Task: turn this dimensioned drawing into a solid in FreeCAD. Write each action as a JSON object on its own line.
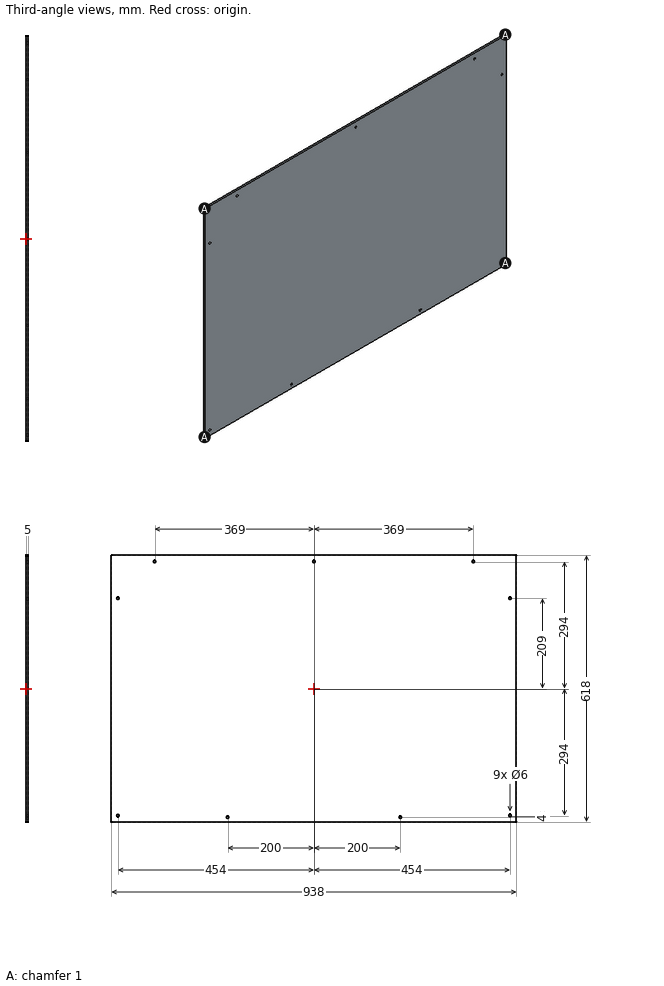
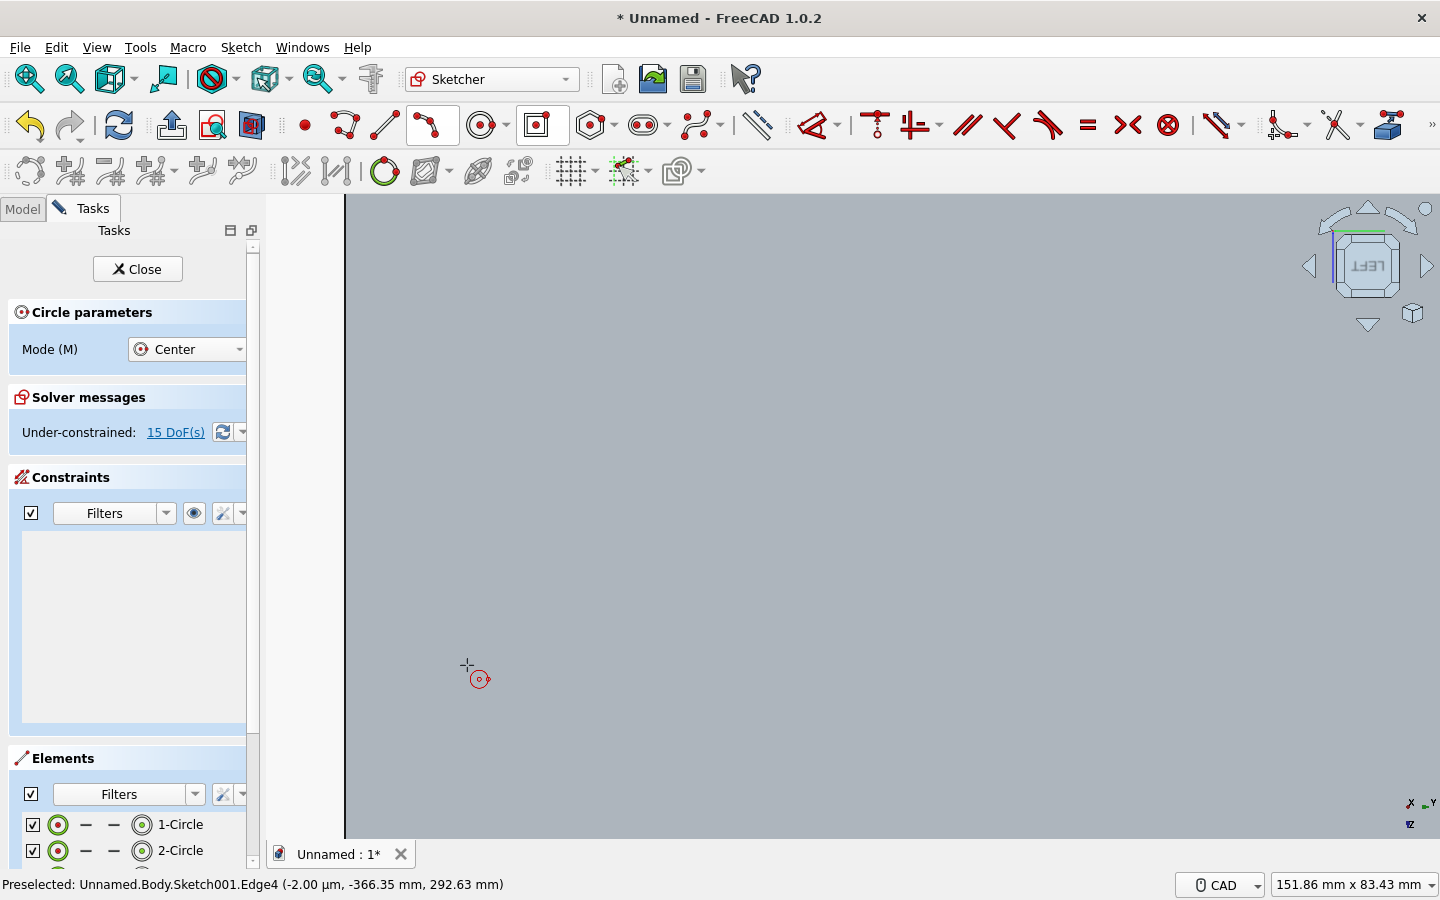
{"action": "scroll", "coordinate": [467, 665], "scroll_direction": "down", "scroll_amount": 12}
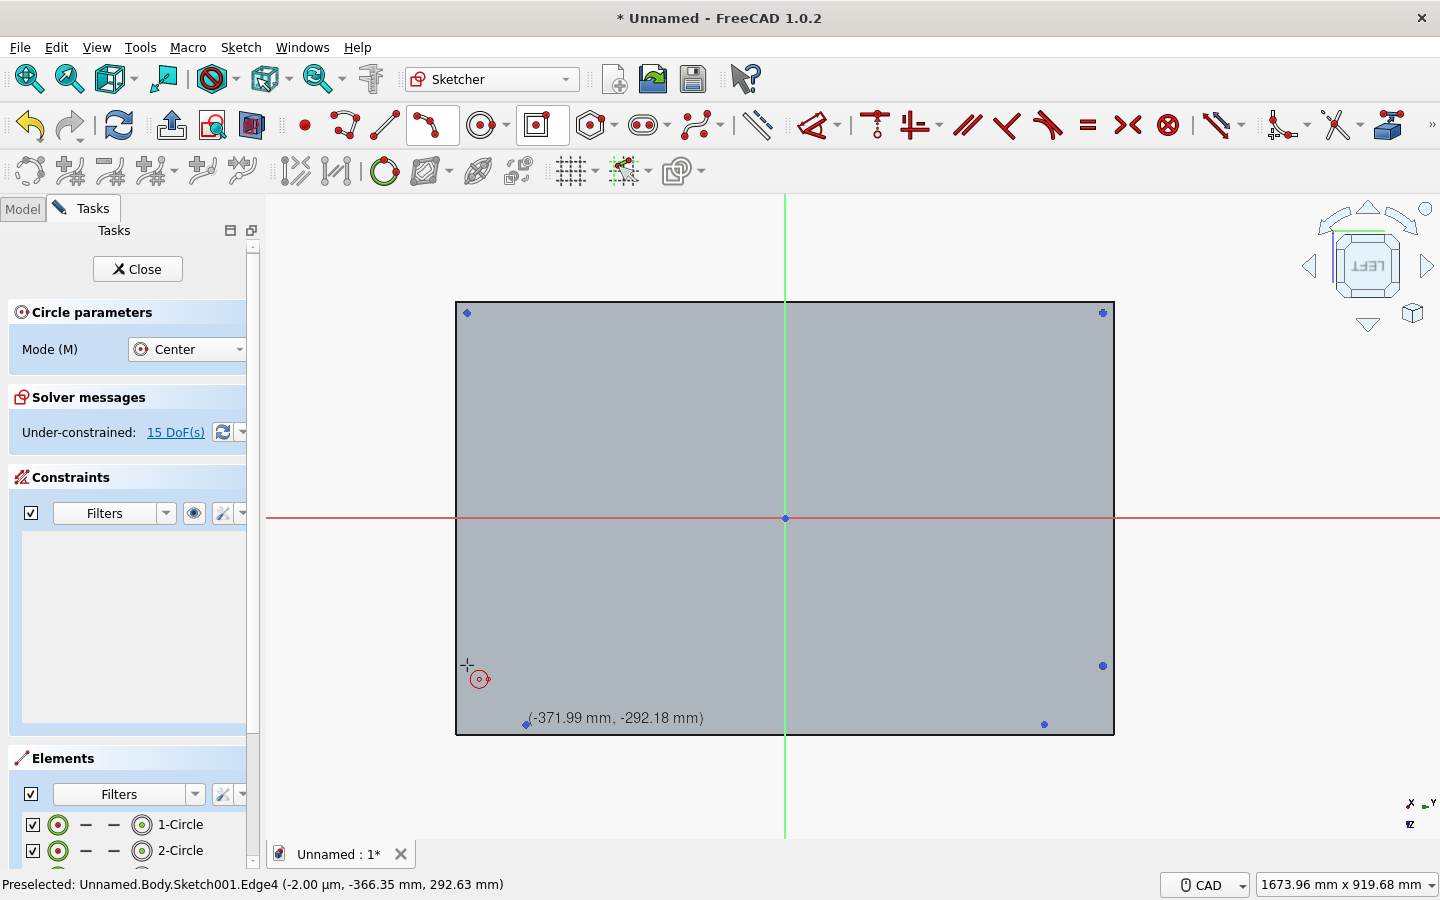
{"action": "left_click", "coordinate": [467, 665]}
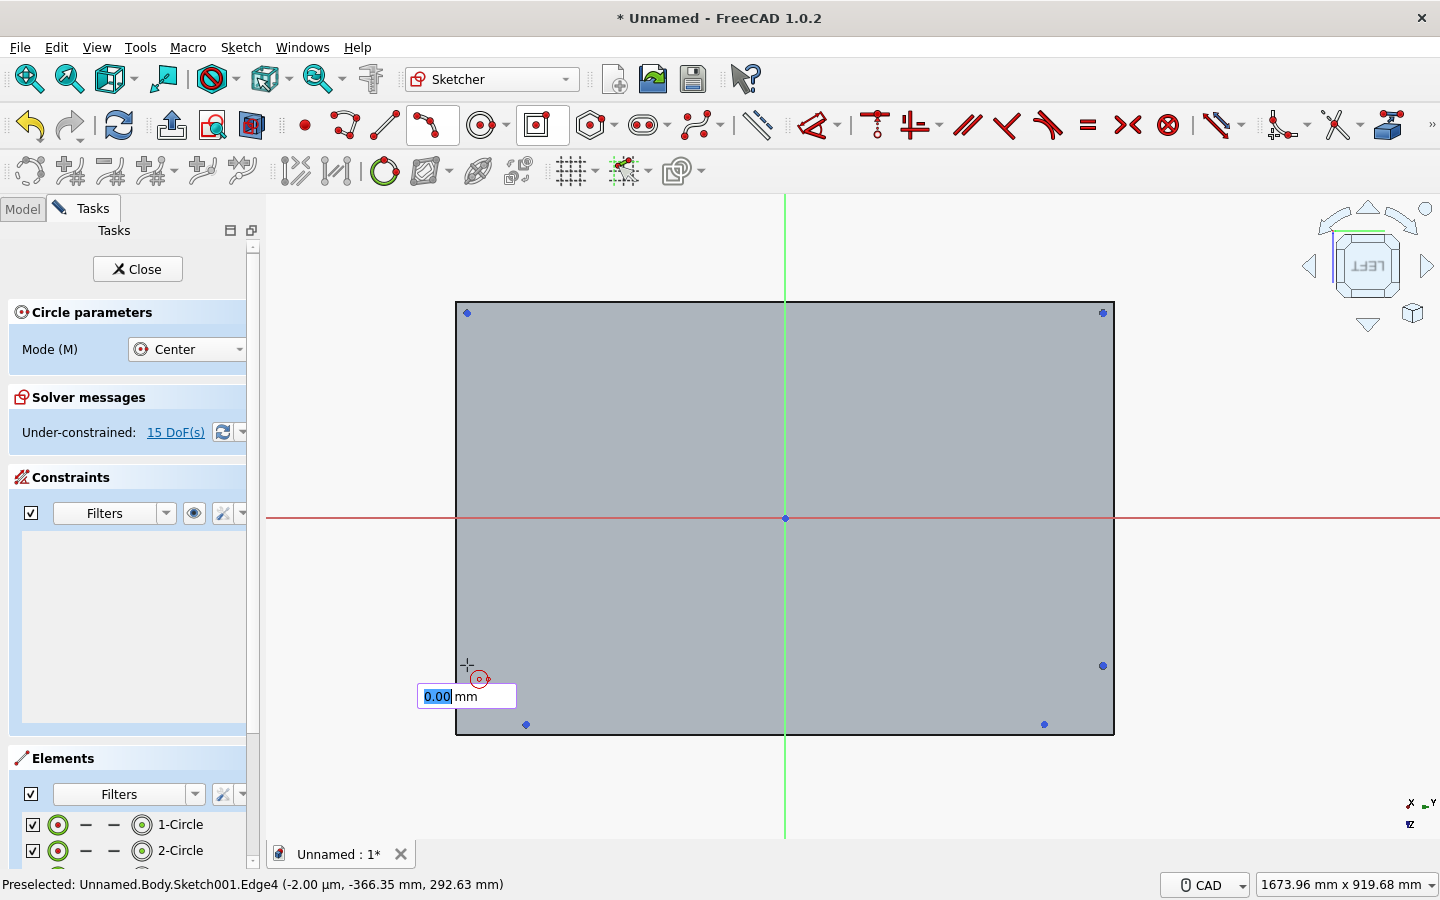
{"action": "scroll", "coordinate": [468, 663], "scroll_direction": "up", "scroll_amount": 11}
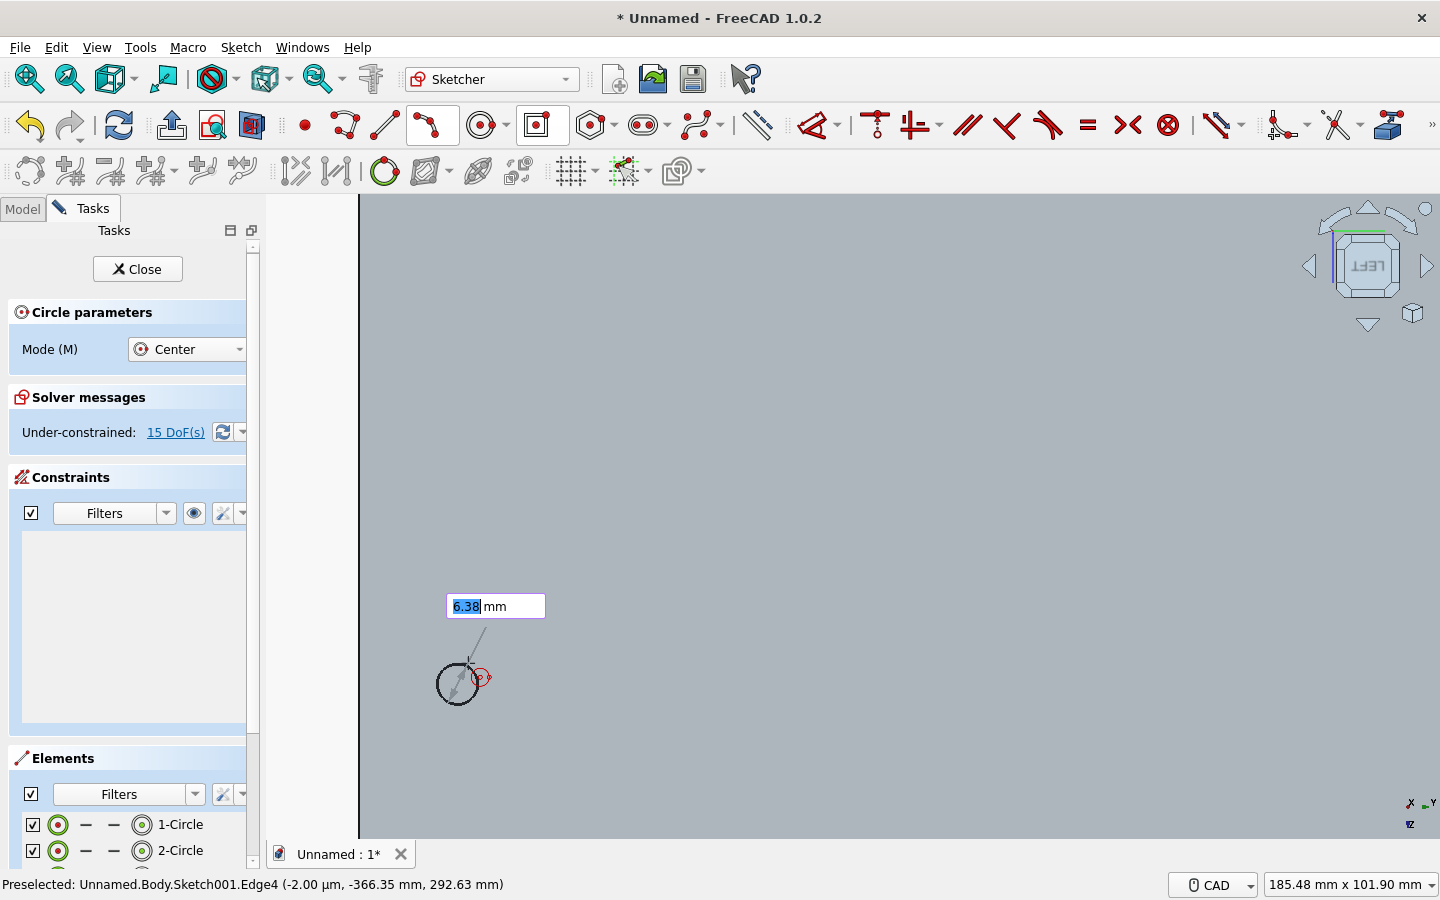
{"action": "left_click", "coordinate": [468, 660]}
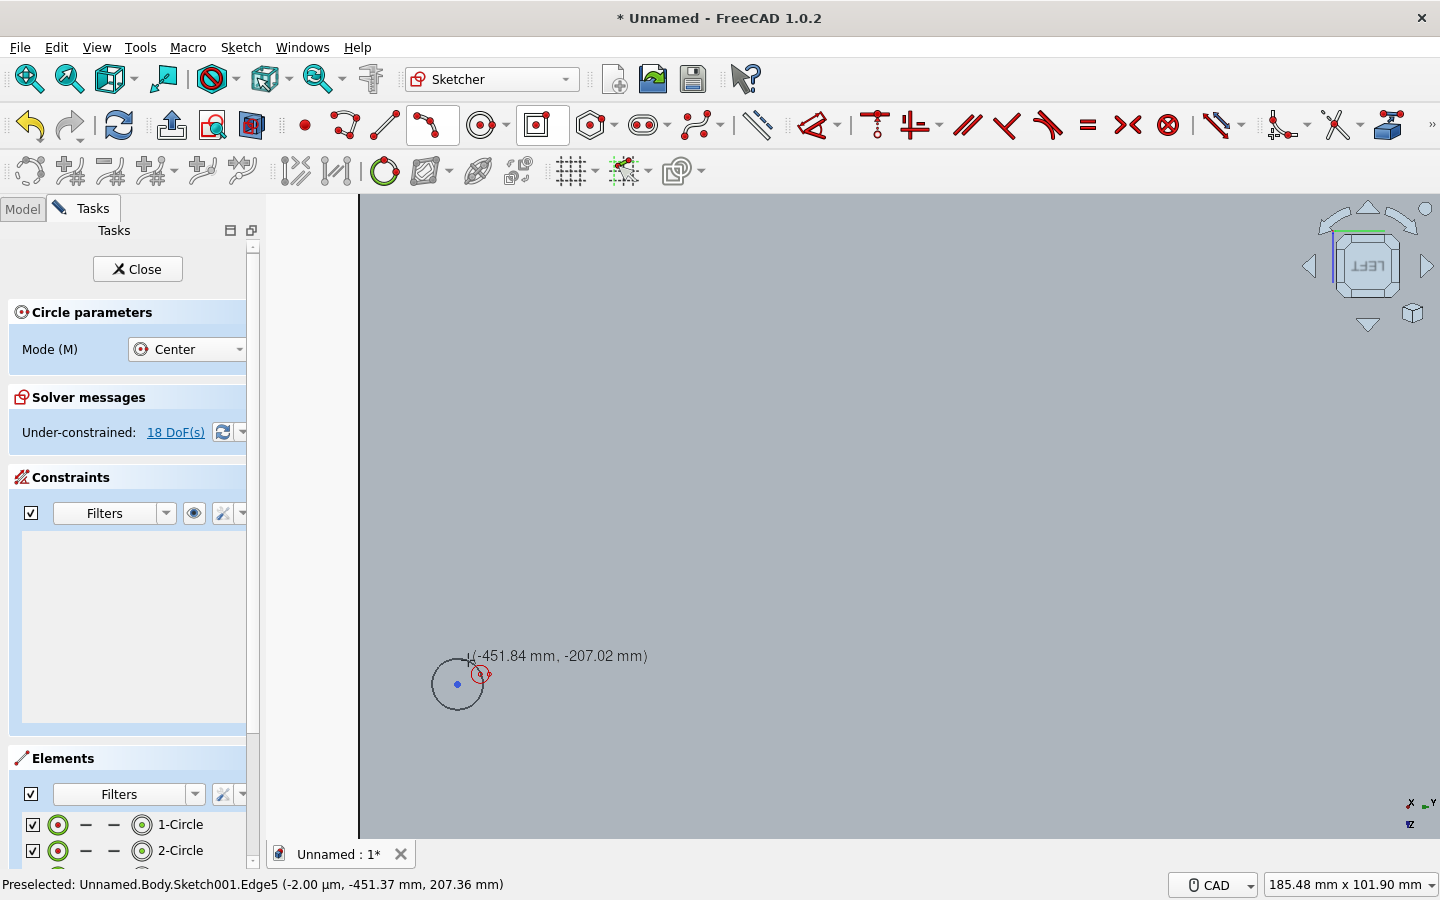
{"action": "scroll", "coordinate": [468, 663], "scroll_direction": "down", "scroll_amount": 11}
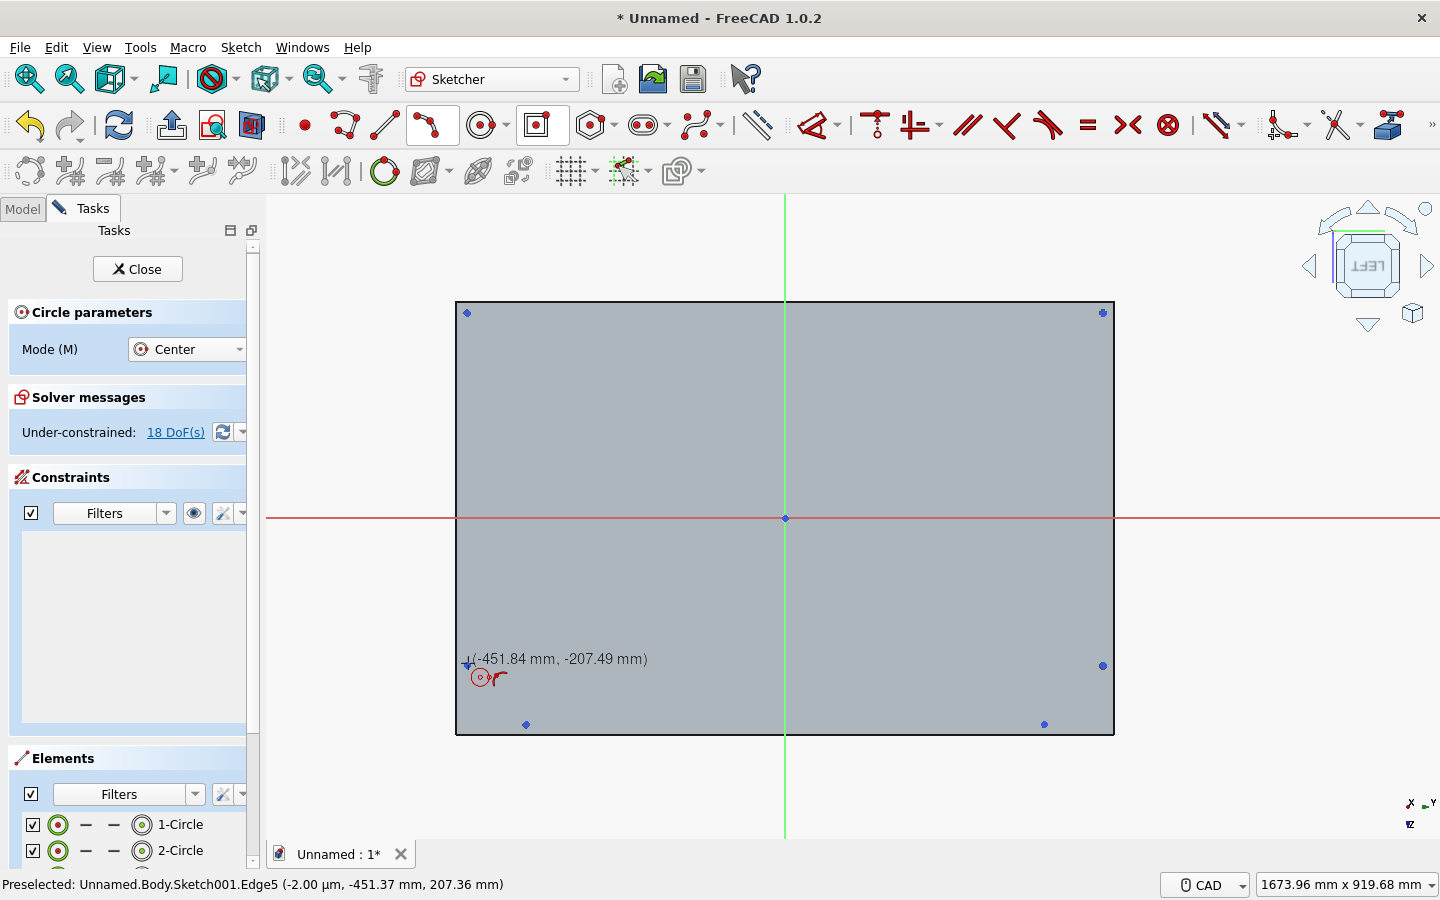
{"action": "scroll", "coordinate": [785, 724], "scroll_direction": "up", "scroll_amount": 12}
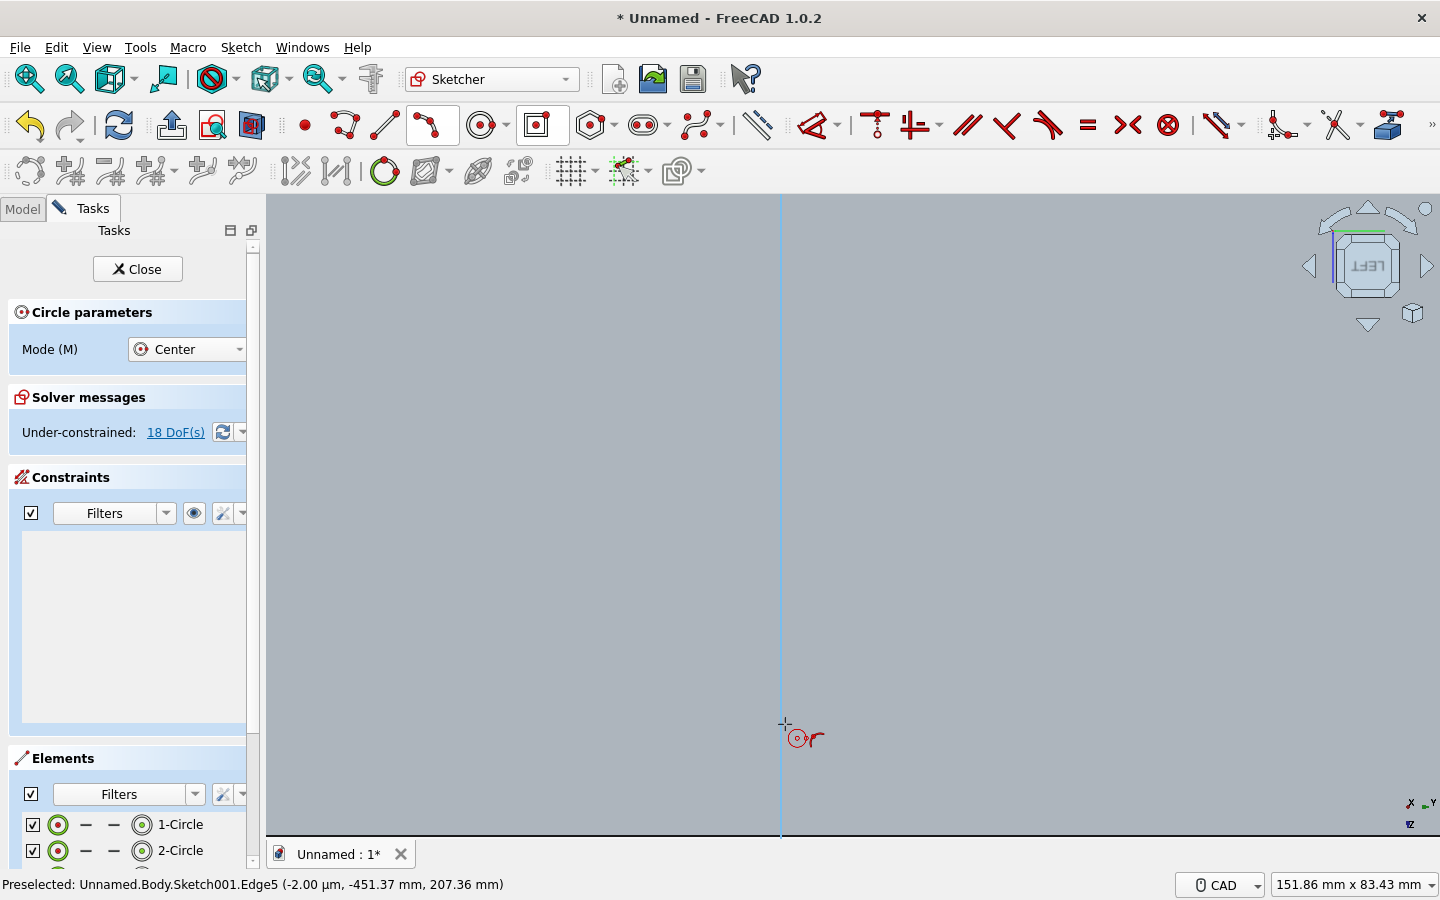
{"action": "scroll", "coordinate": [785, 724], "scroll_direction": "down", "scroll_amount": 12}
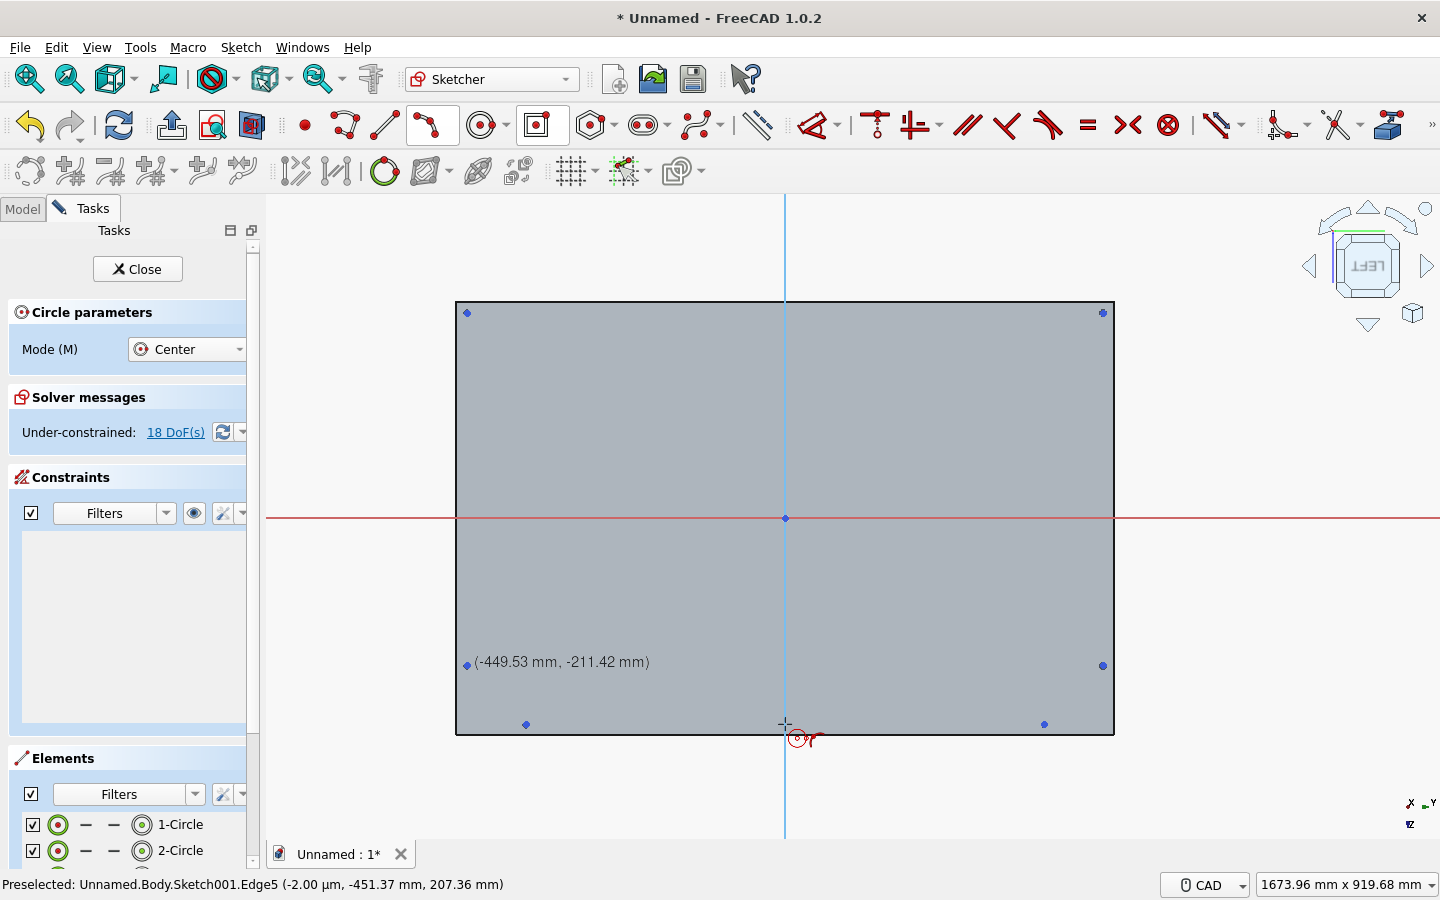
{"action": "left_click", "coordinate": [785, 724]}